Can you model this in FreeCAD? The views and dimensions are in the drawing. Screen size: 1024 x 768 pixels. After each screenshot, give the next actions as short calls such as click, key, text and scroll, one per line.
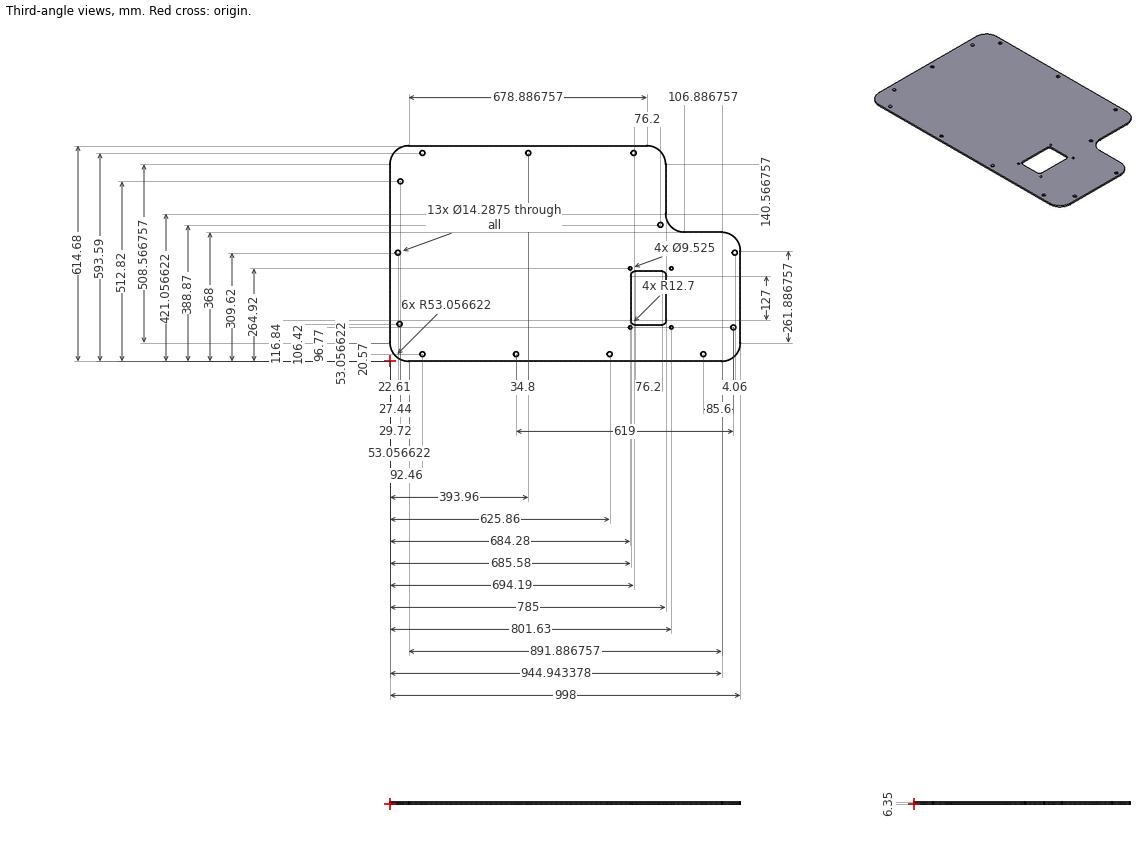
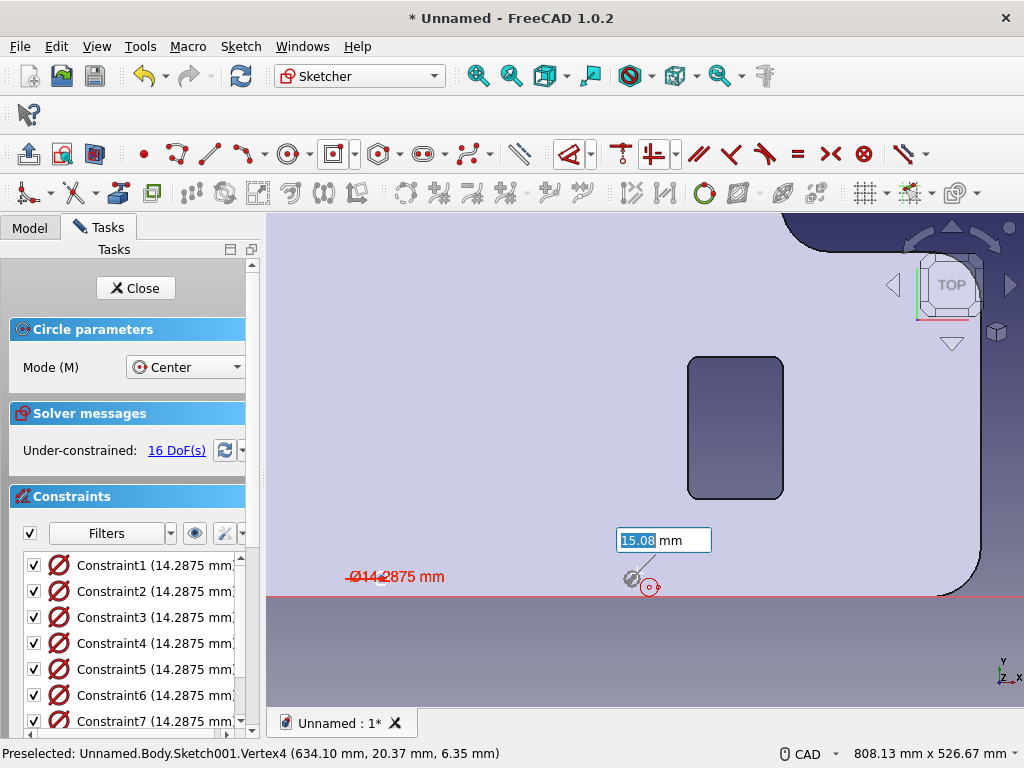
text(14.2875)
key(Return)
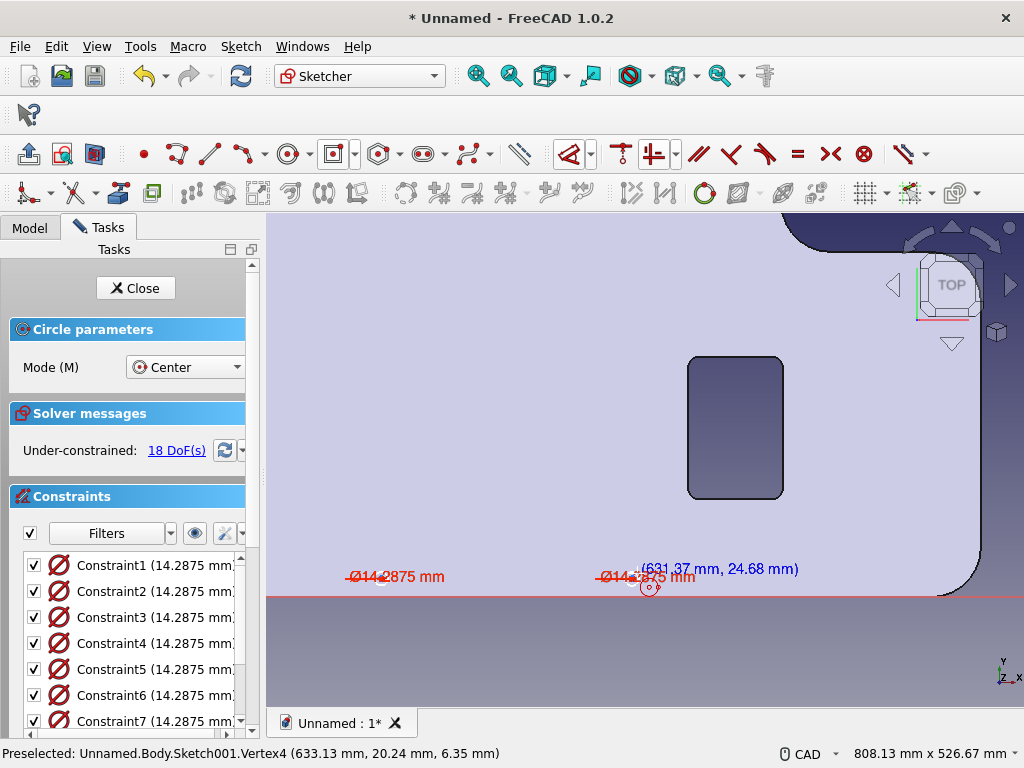
scroll(632, 578, down, 4)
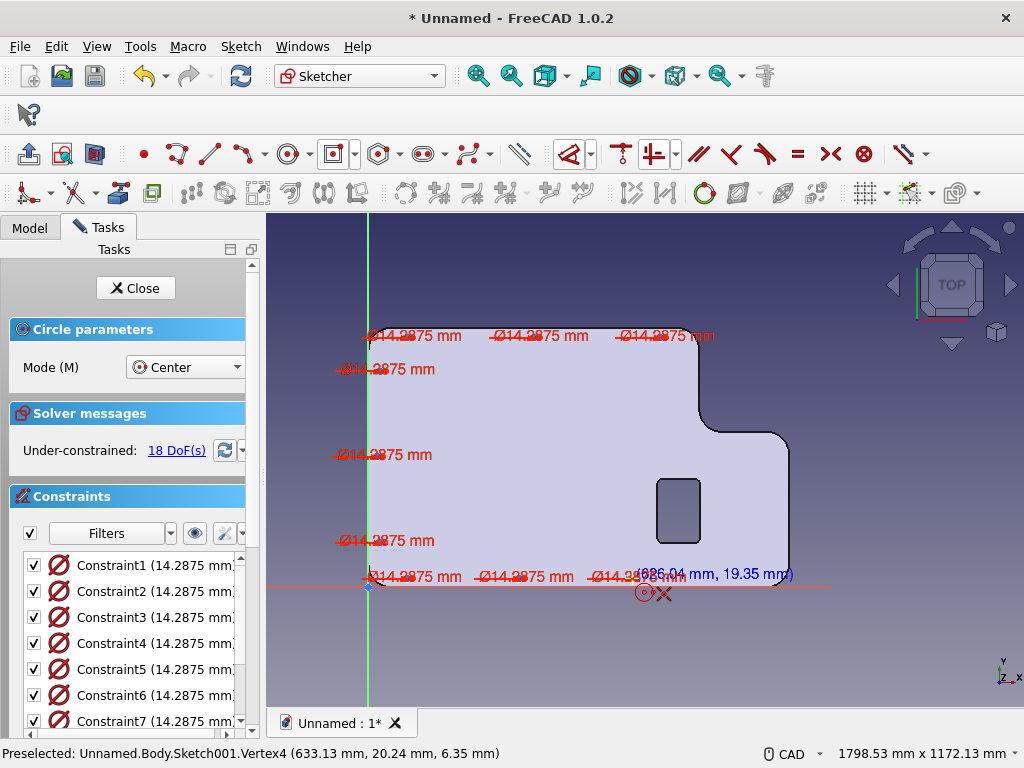
scroll(745, 578, up, 11)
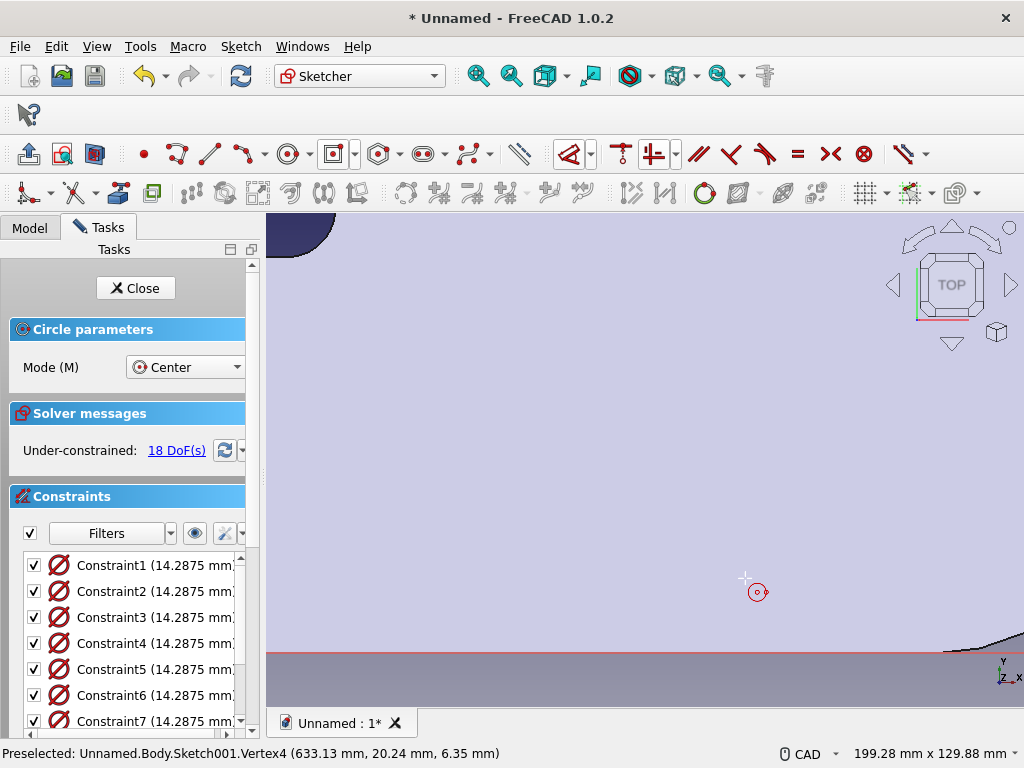
scroll(745, 578, down, 11)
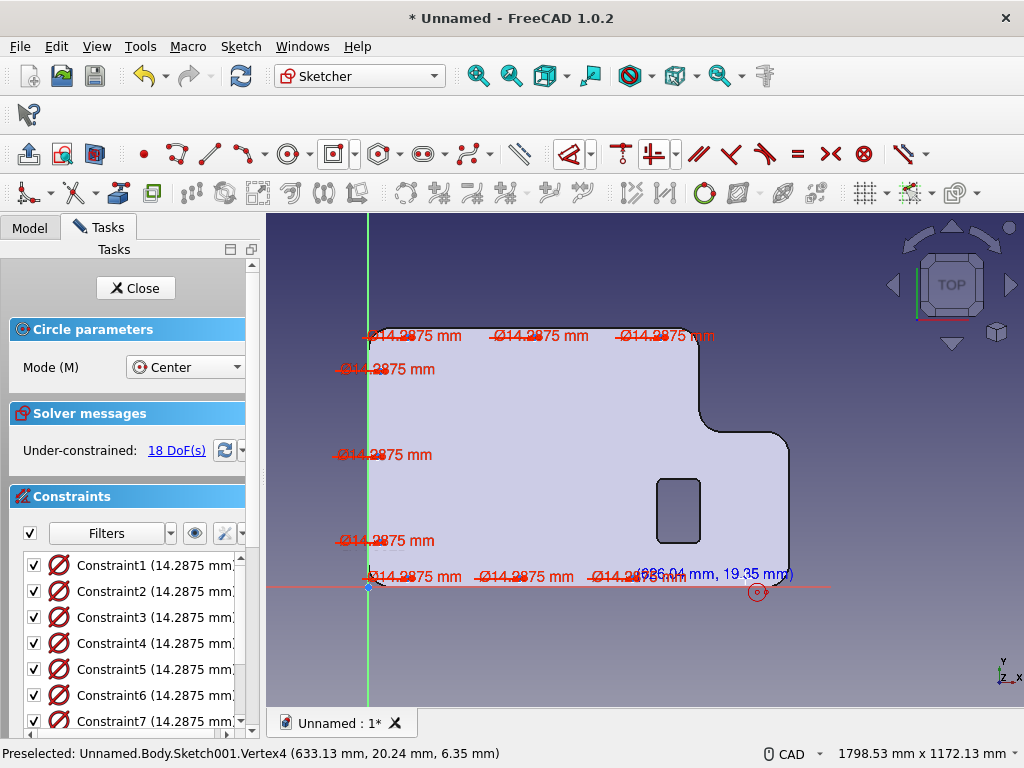
scroll(745, 578, up, 4)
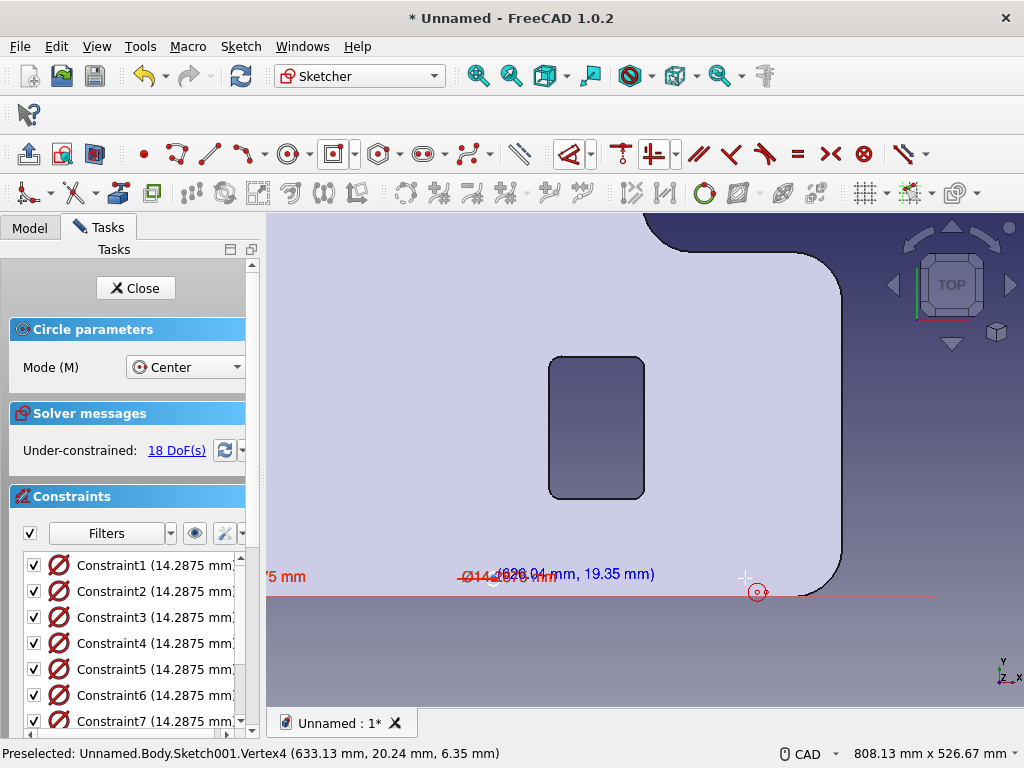
click(743, 578)
move(748, 573)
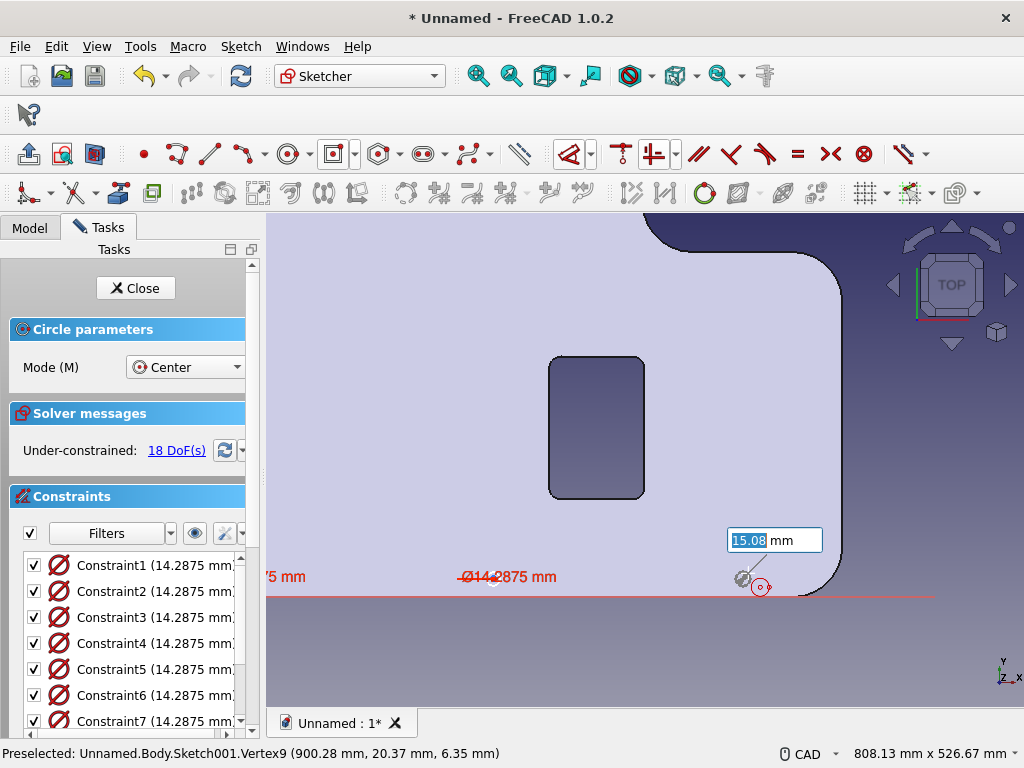
text(14.2875)
key(Return)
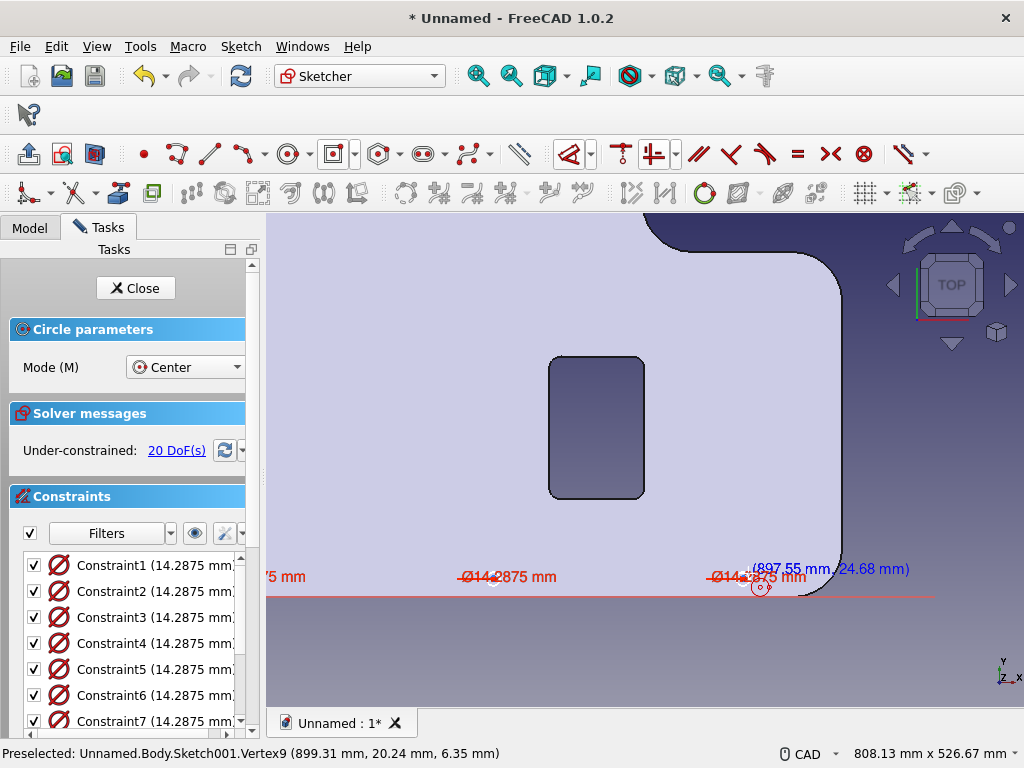
scroll(824, 506, up, 7)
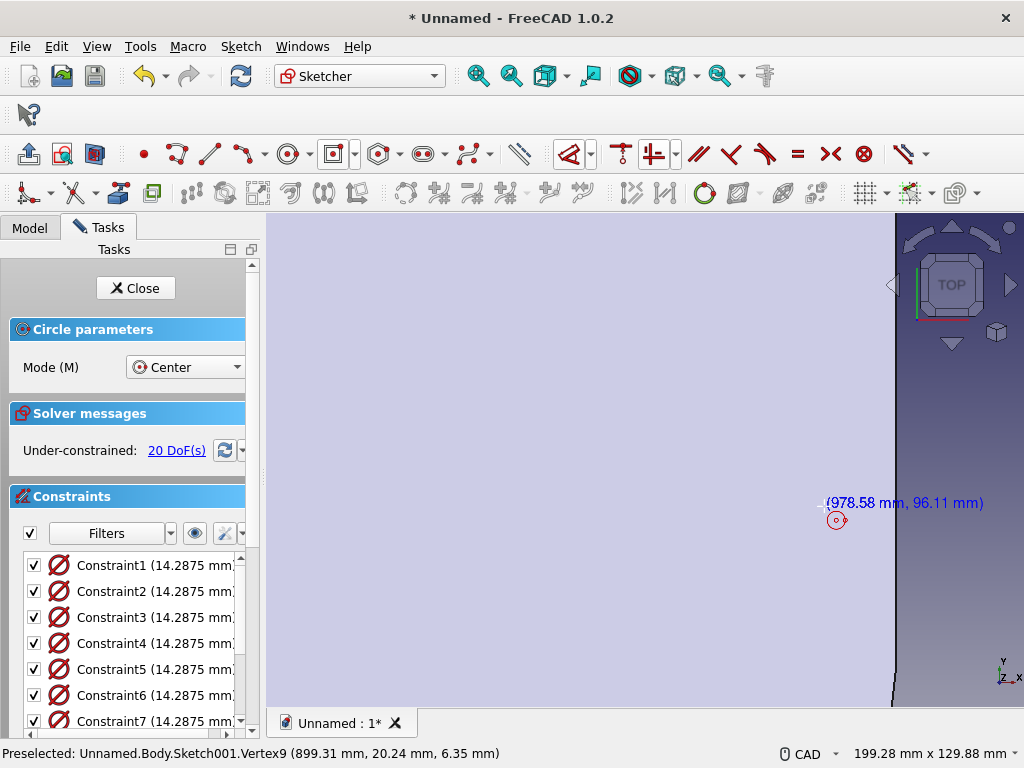
scroll(775, 551, down, 11)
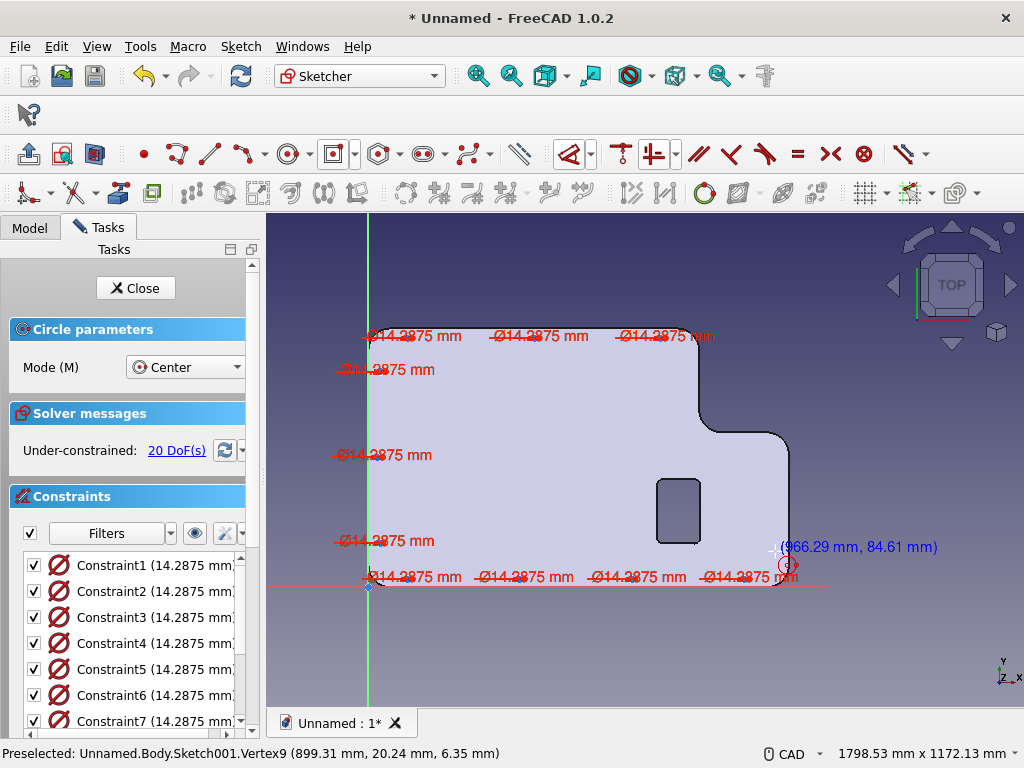
click(781, 547)
move(783, 544)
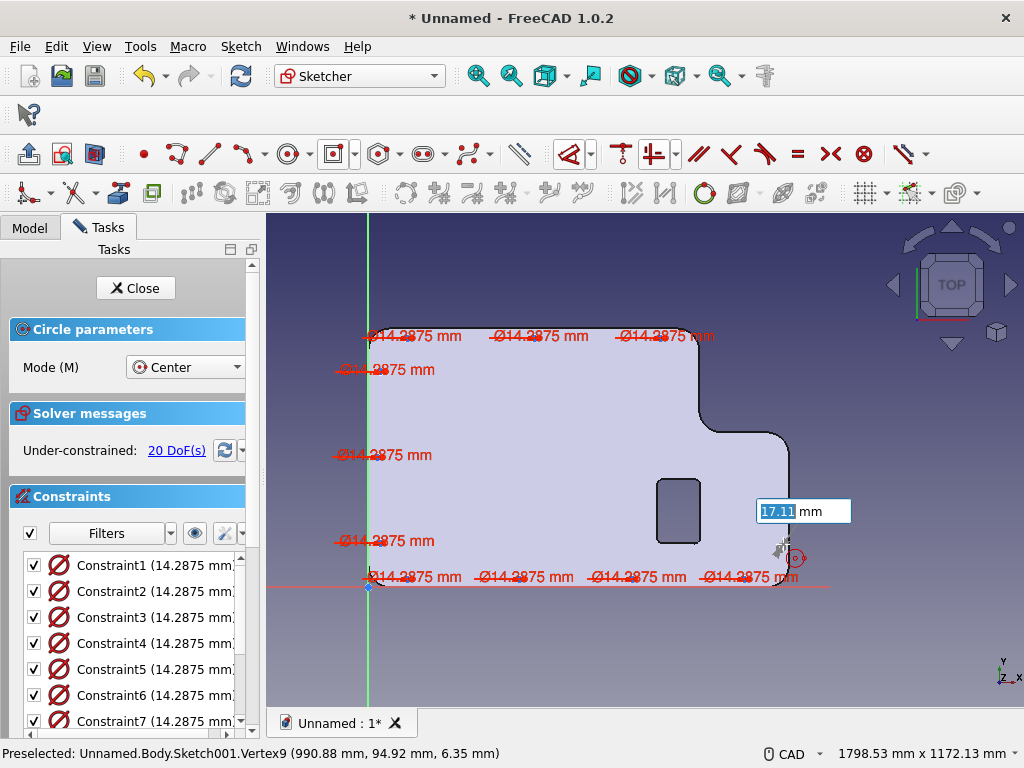
text(14.2875)
key(Return)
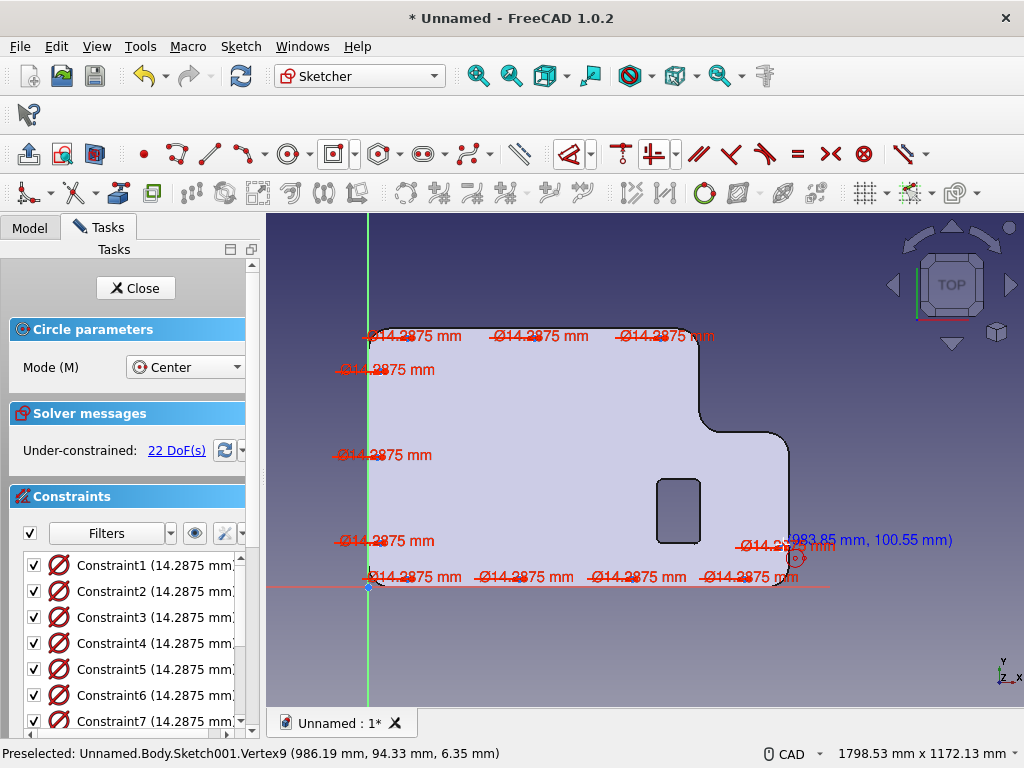
scroll(782, 457, up, 11)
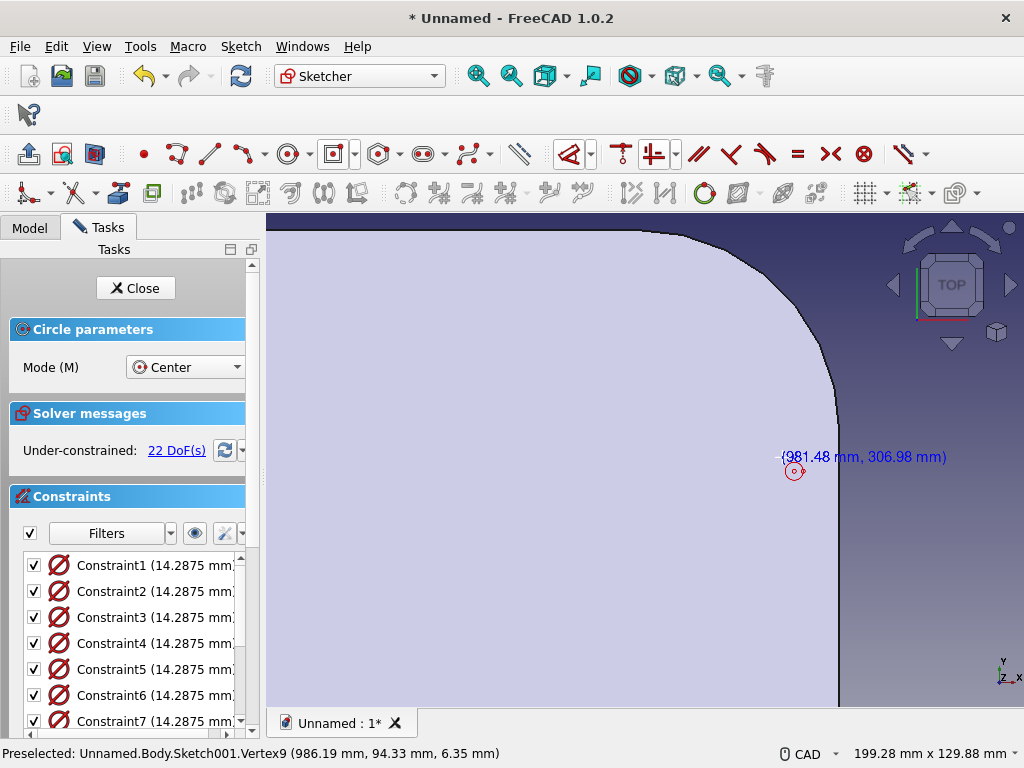
scroll(782, 457, down, 11)